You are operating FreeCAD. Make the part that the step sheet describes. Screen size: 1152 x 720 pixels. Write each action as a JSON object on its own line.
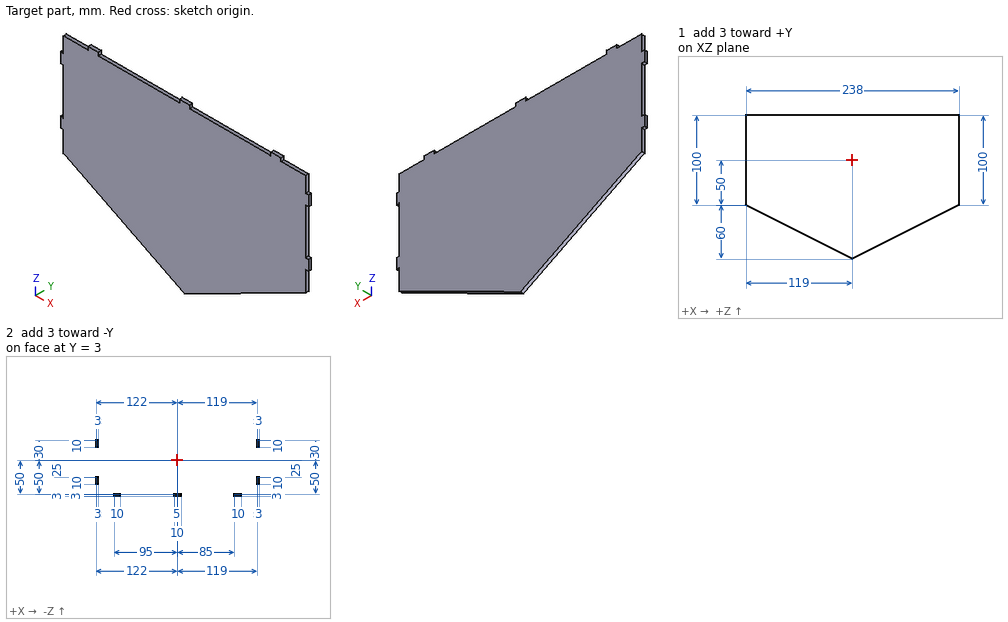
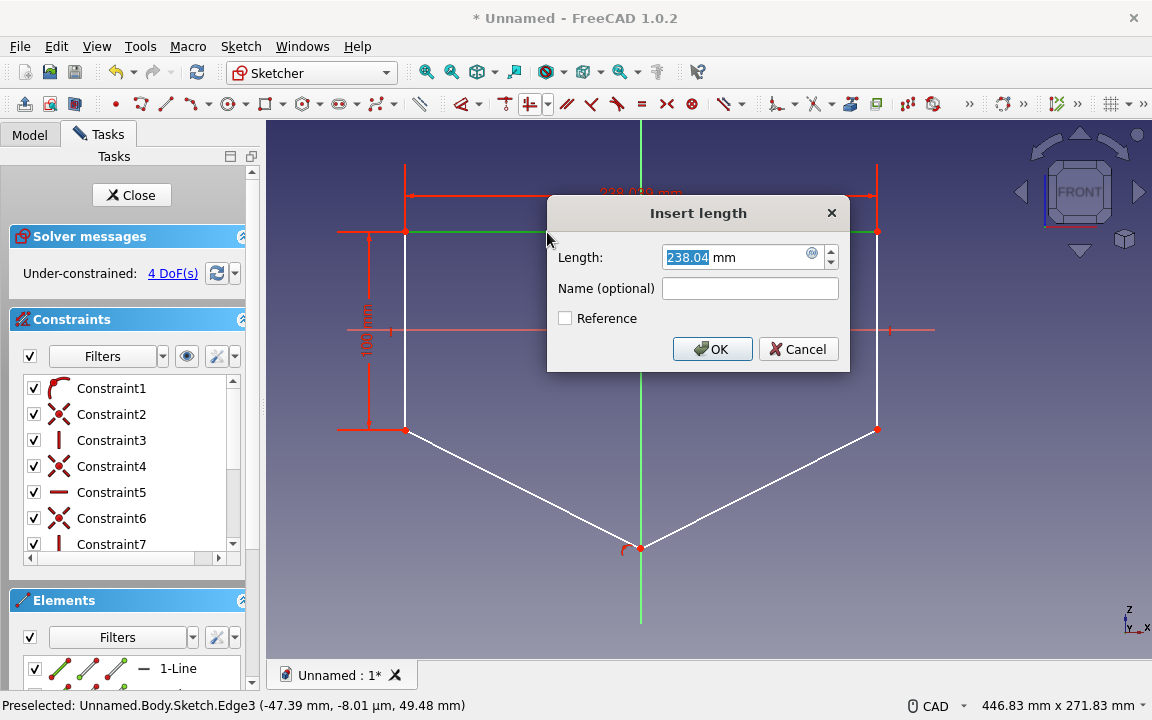
{"action": "type", "text": "238"}
{"action": "key", "text": "Return"}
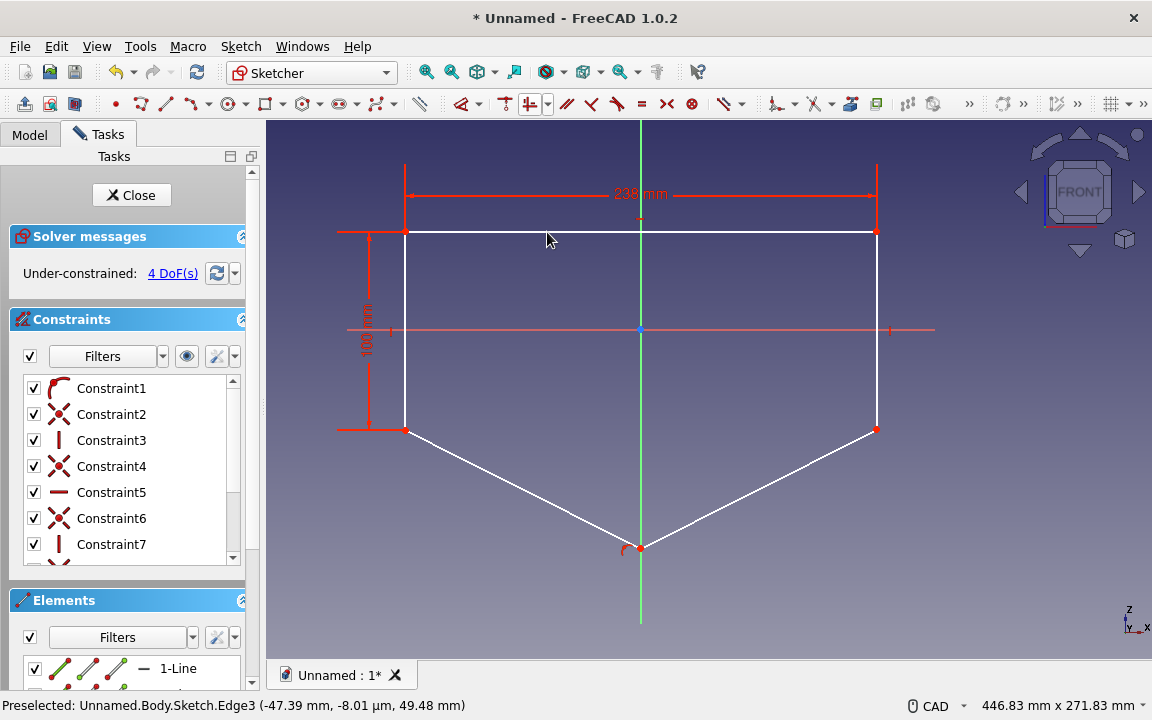
{"action": "left_click", "coordinate": [877, 291]}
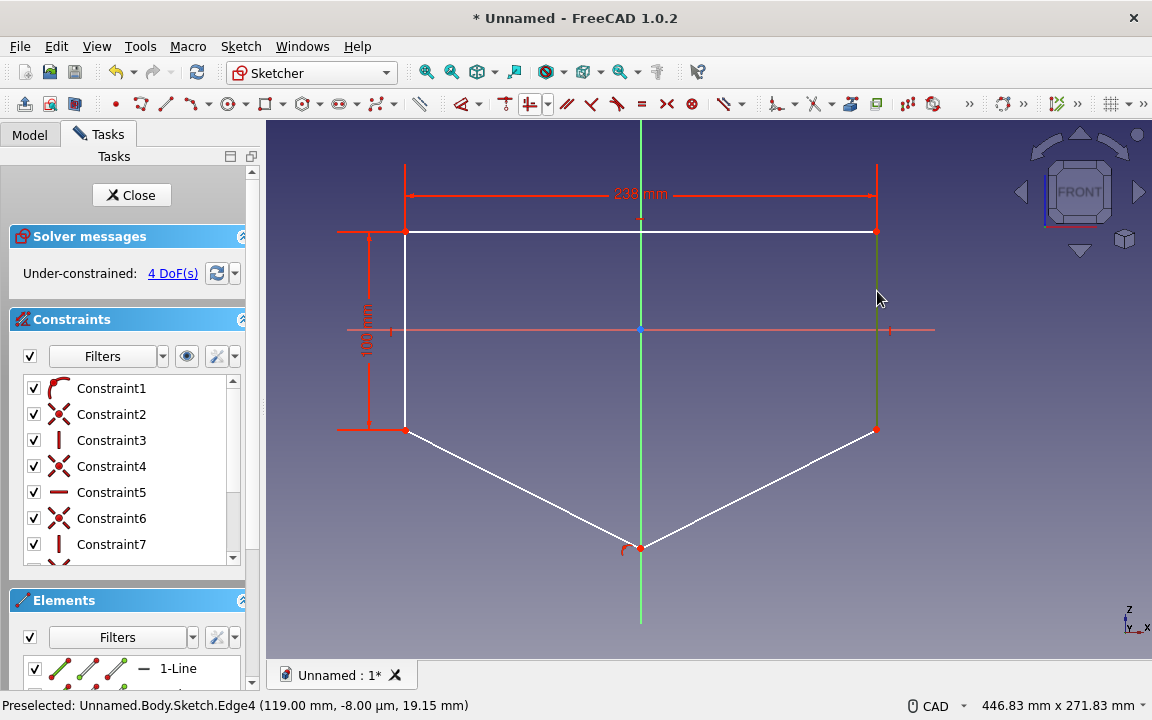
{"action": "left_click", "coordinate": [478, 104]}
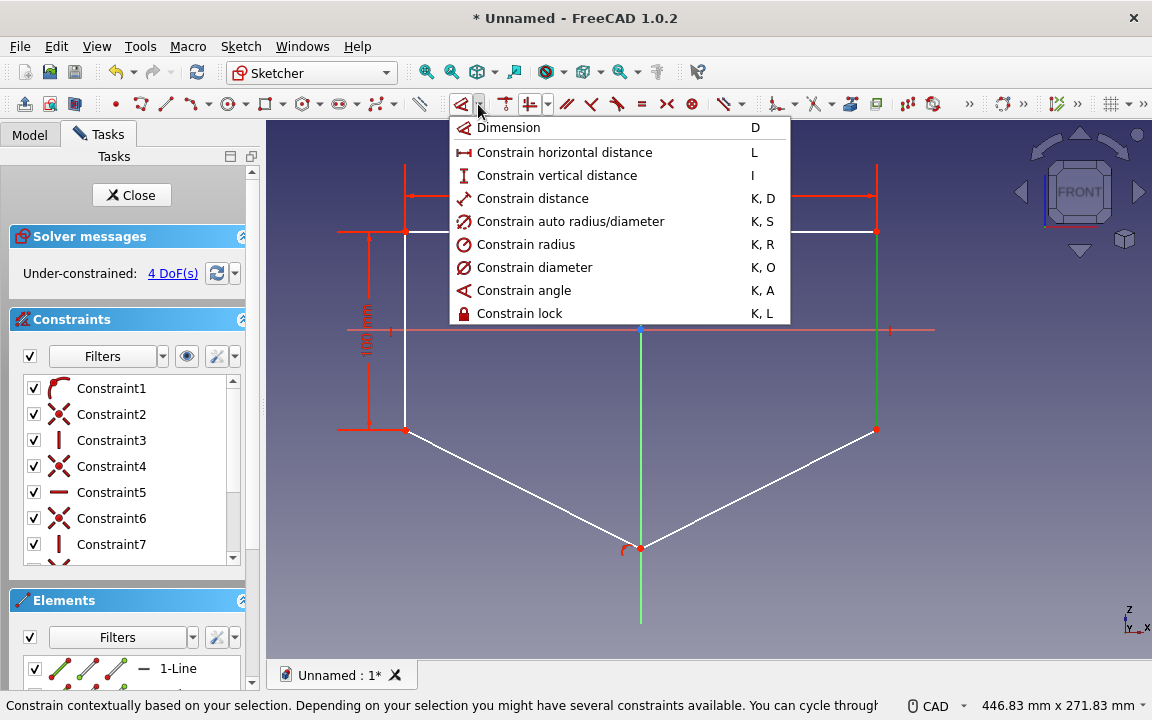
{"action": "left_click", "coordinate": [620, 176]}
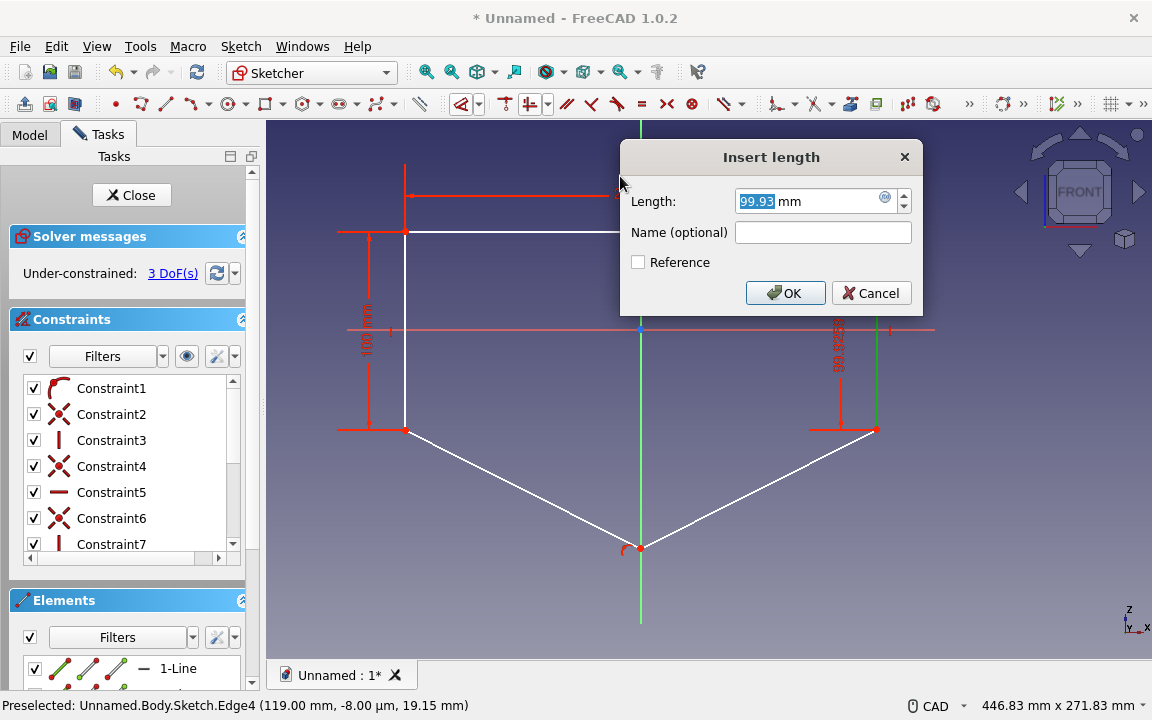
{"action": "type", "text": "100"}
{"action": "key", "text": "Return"}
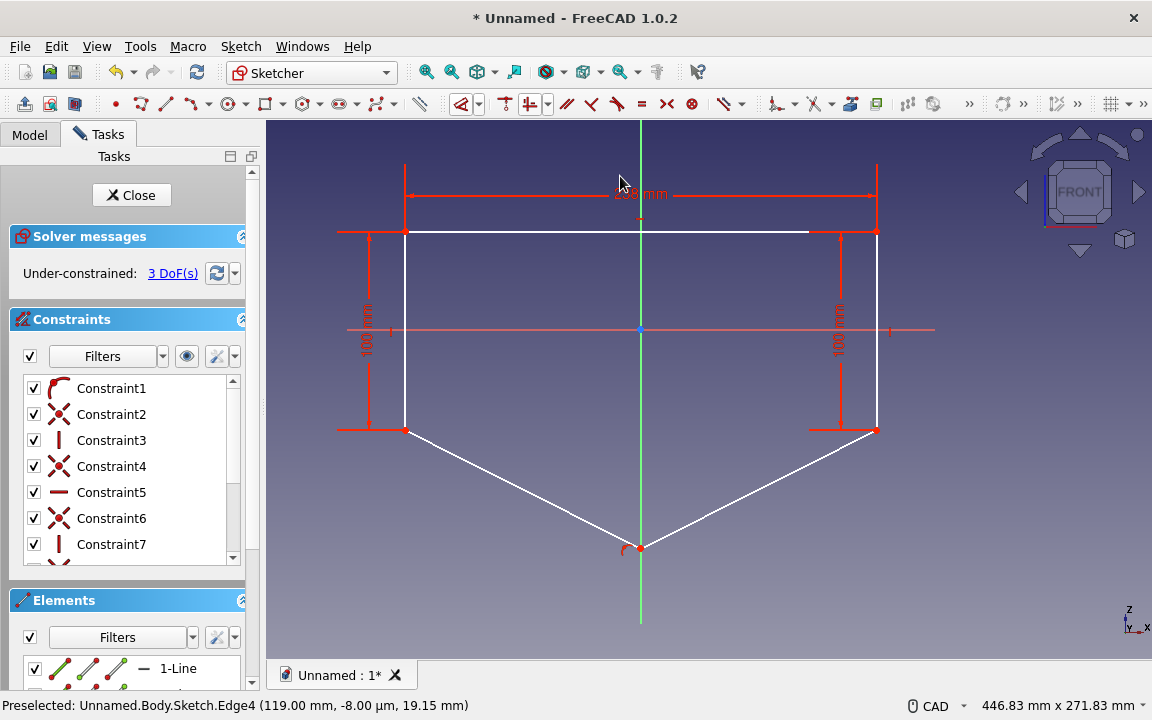
{"action": "left_click", "coordinate": [405, 430]}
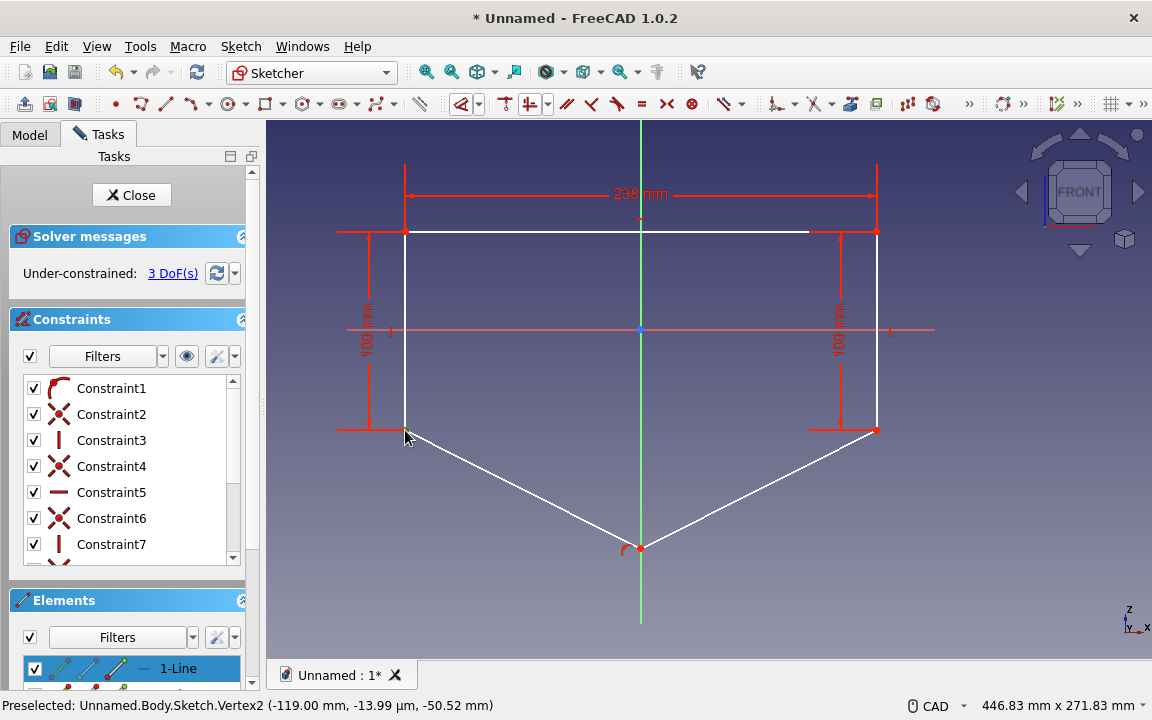
{"action": "key", "text": "i"}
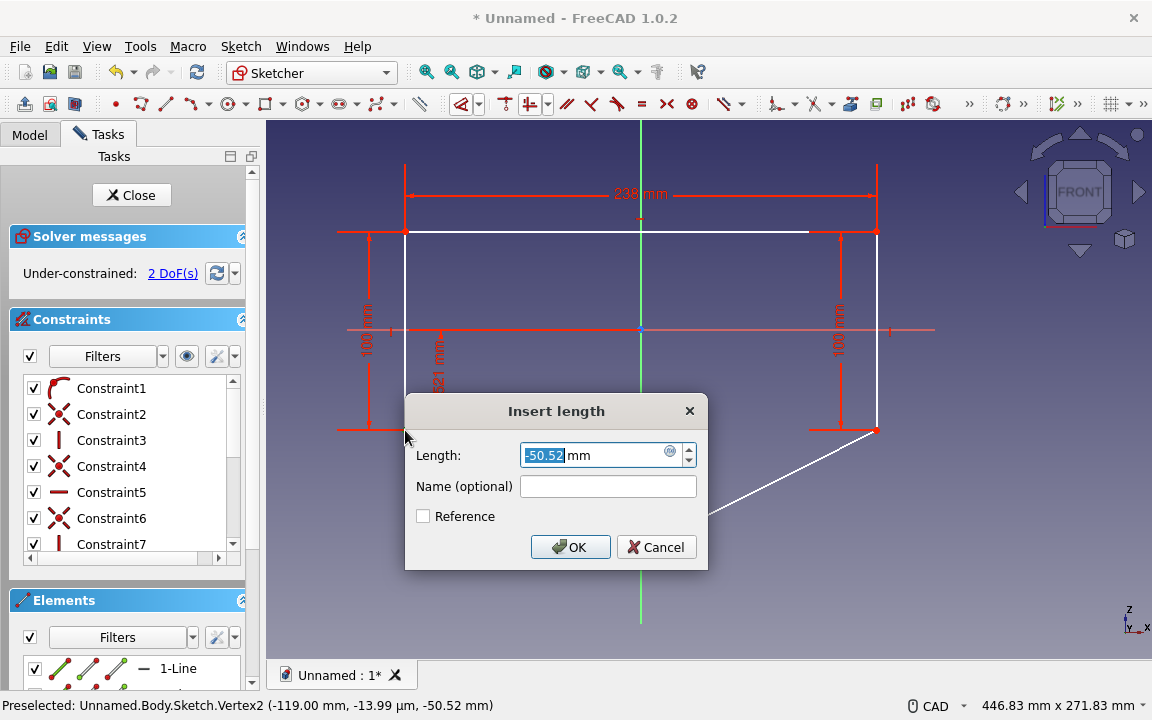
{"action": "type", "text": "-50"}
{"action": "key", "text": "Return"}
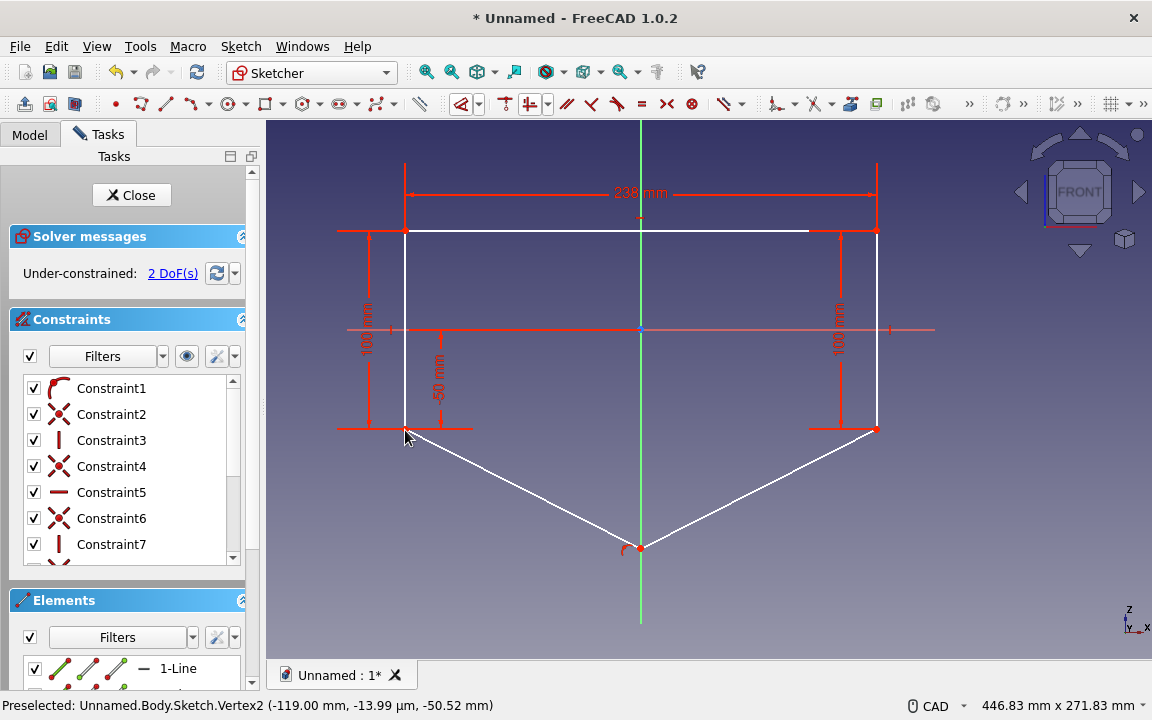
{"action": "left_click", "coordinate": [570, 513]}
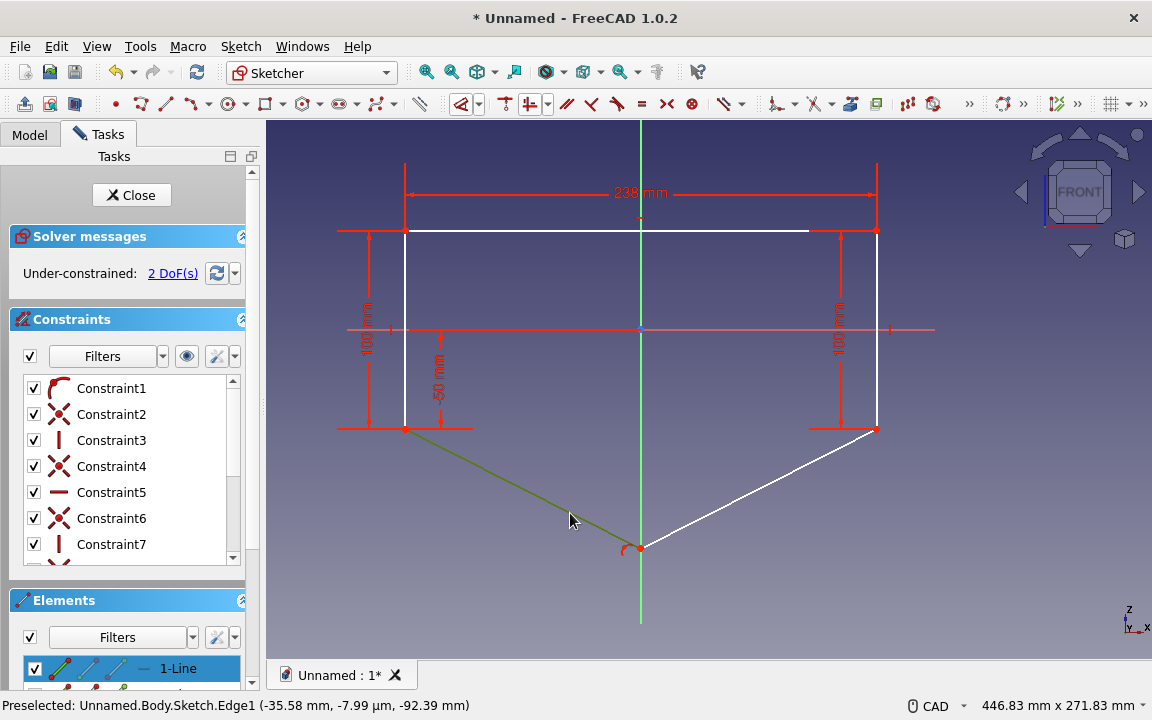
{"action": "key", "text": "i"}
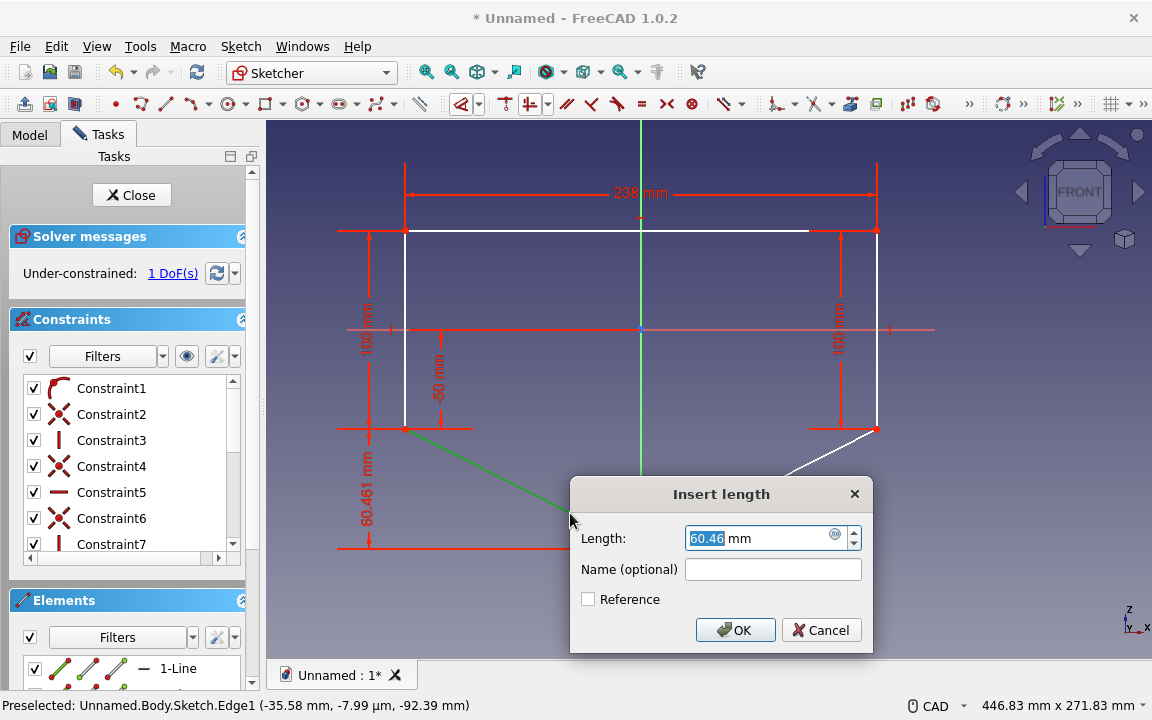
{"action": "type", "text": "60"}
{"action": "key", "text": "Return"}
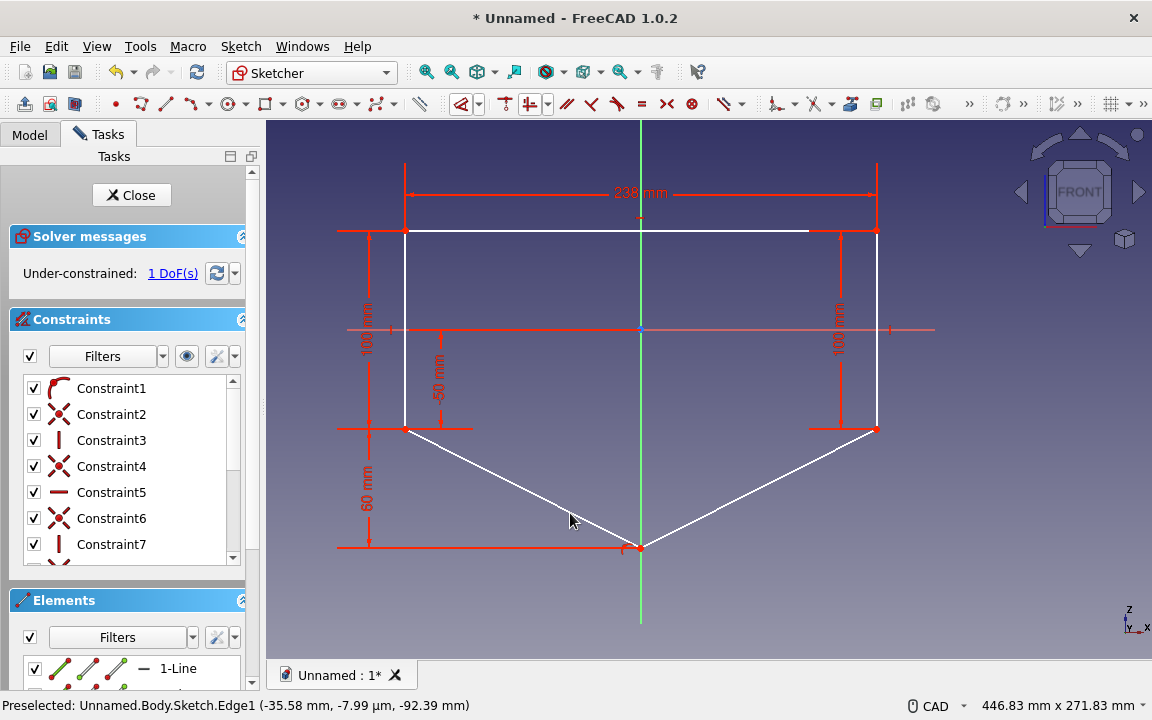
{"action": "left_click", "coordinate": [405, 429]}